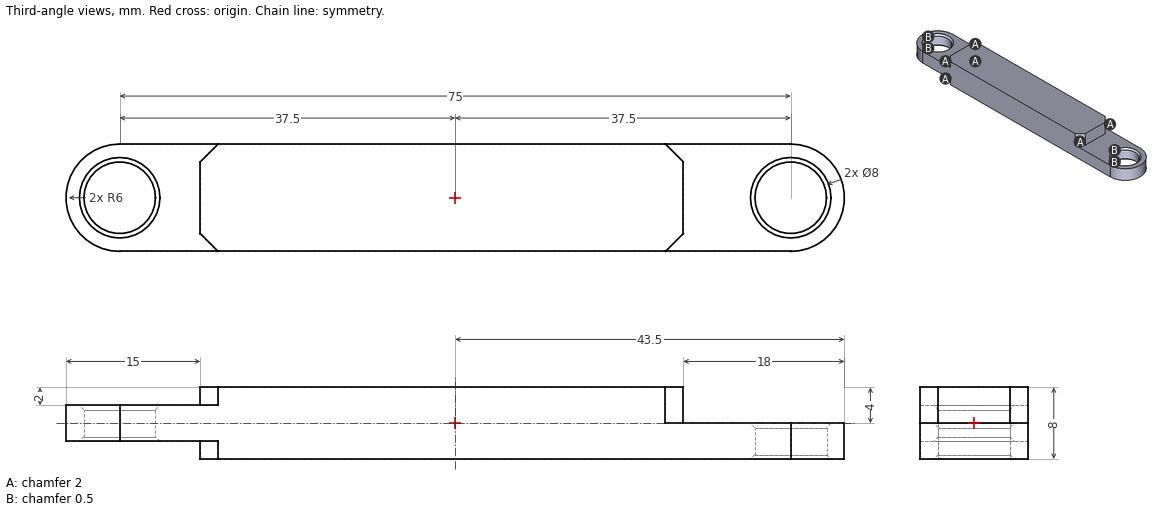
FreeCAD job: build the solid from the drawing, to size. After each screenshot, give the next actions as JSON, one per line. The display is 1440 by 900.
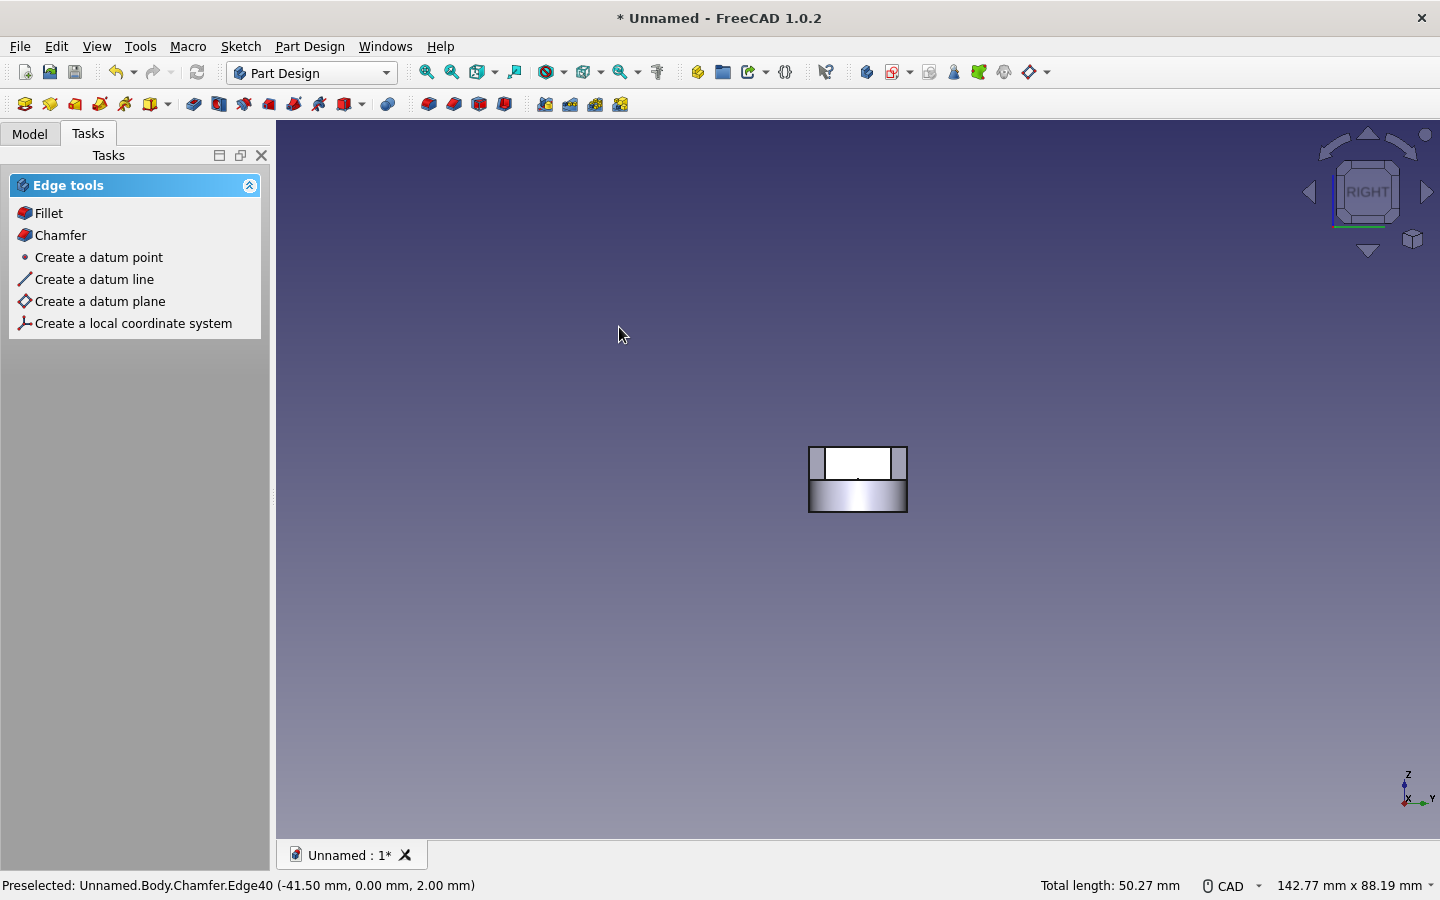
{"action": "left_click", "coordinate": [427, 72]}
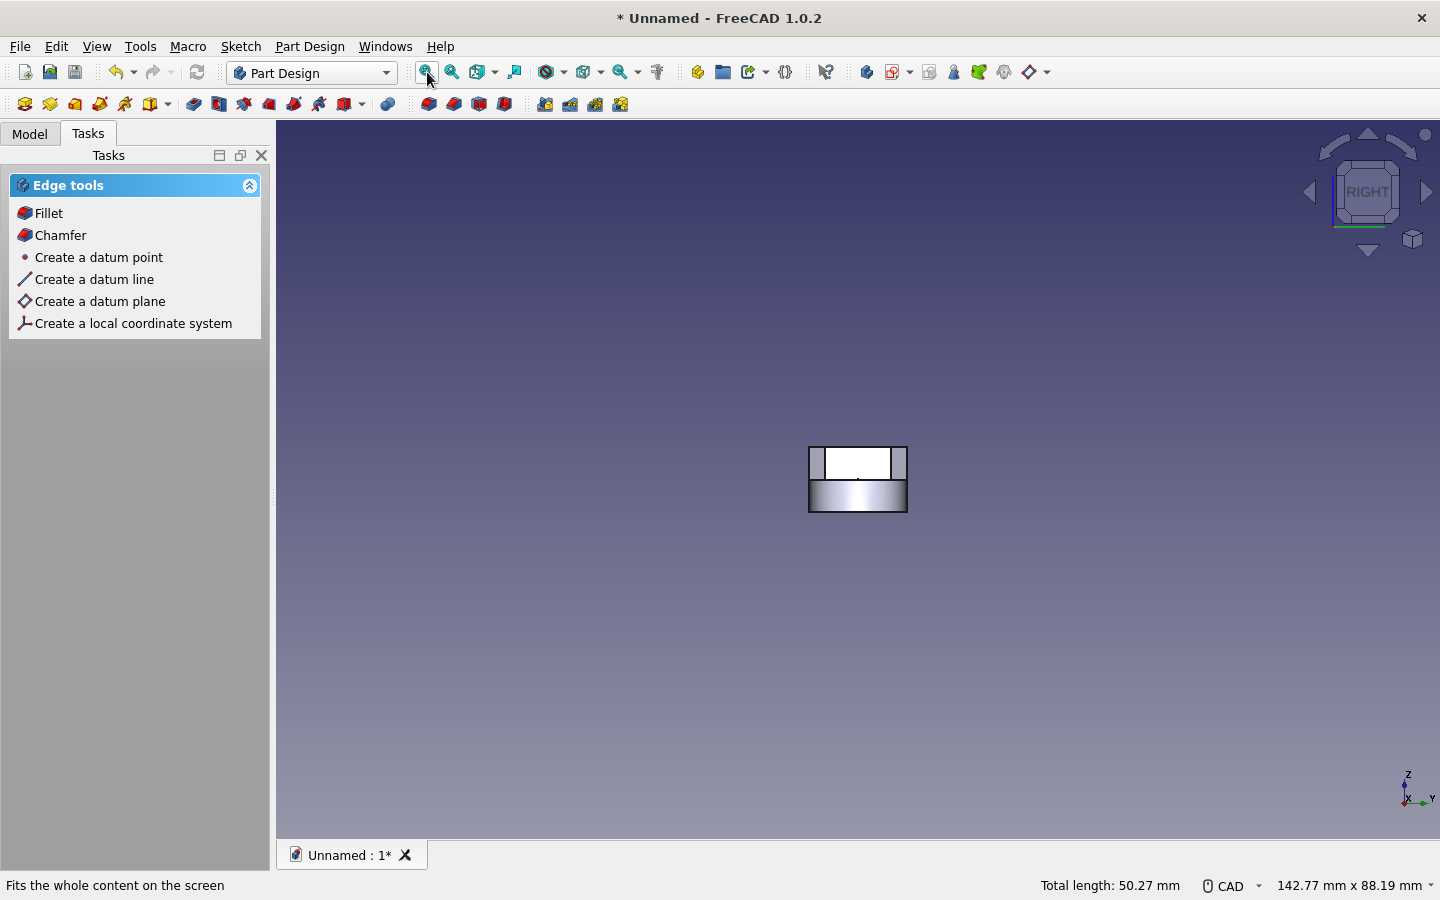
{"action": "key", "text": "5"}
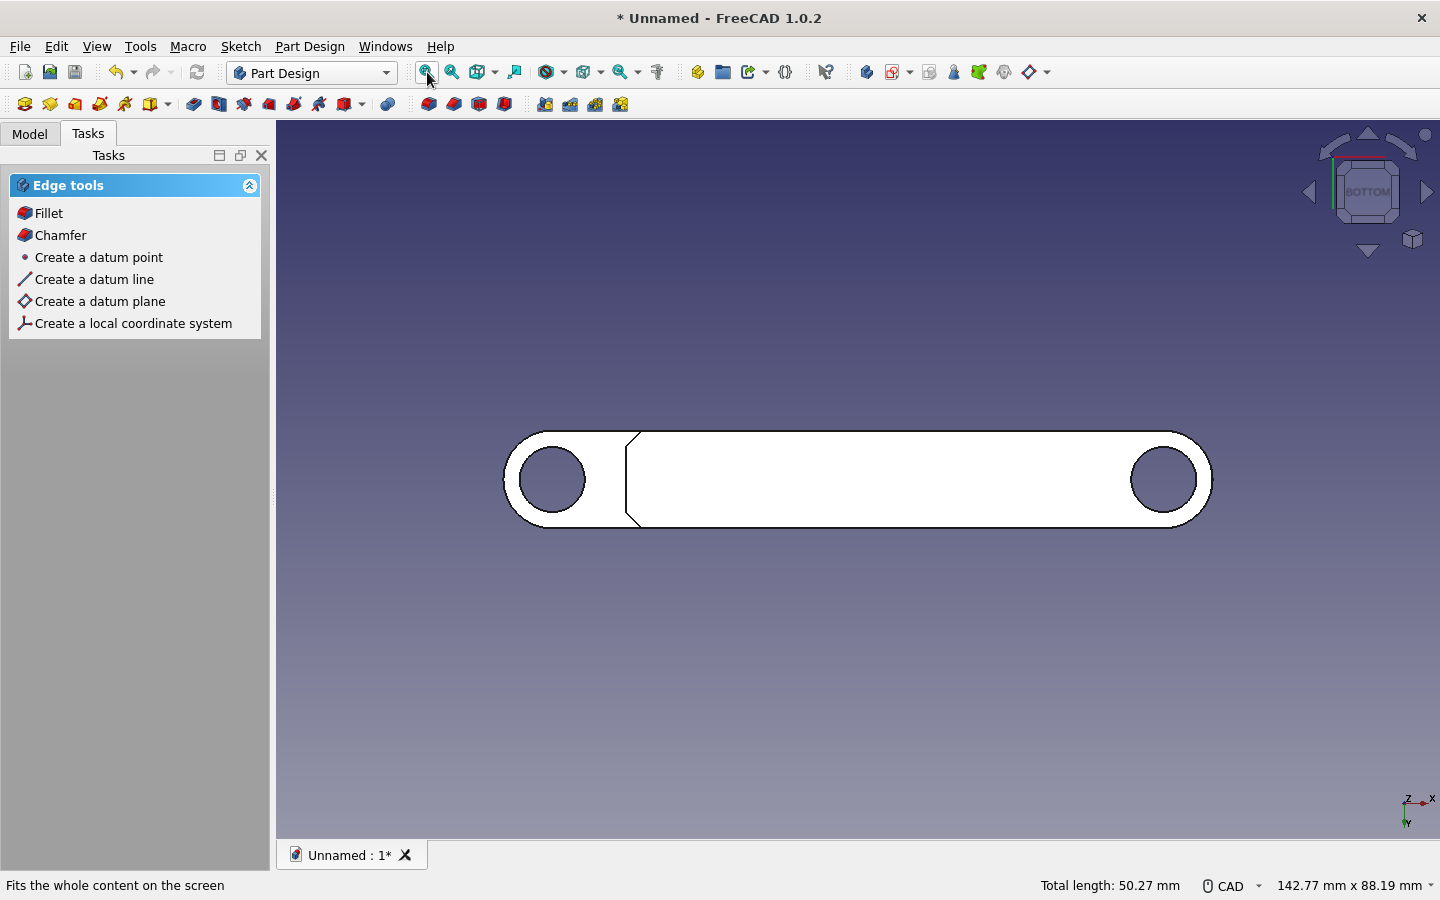
{"action": "left_click", "coordinate": [1131, 478], "text": "ctrl"}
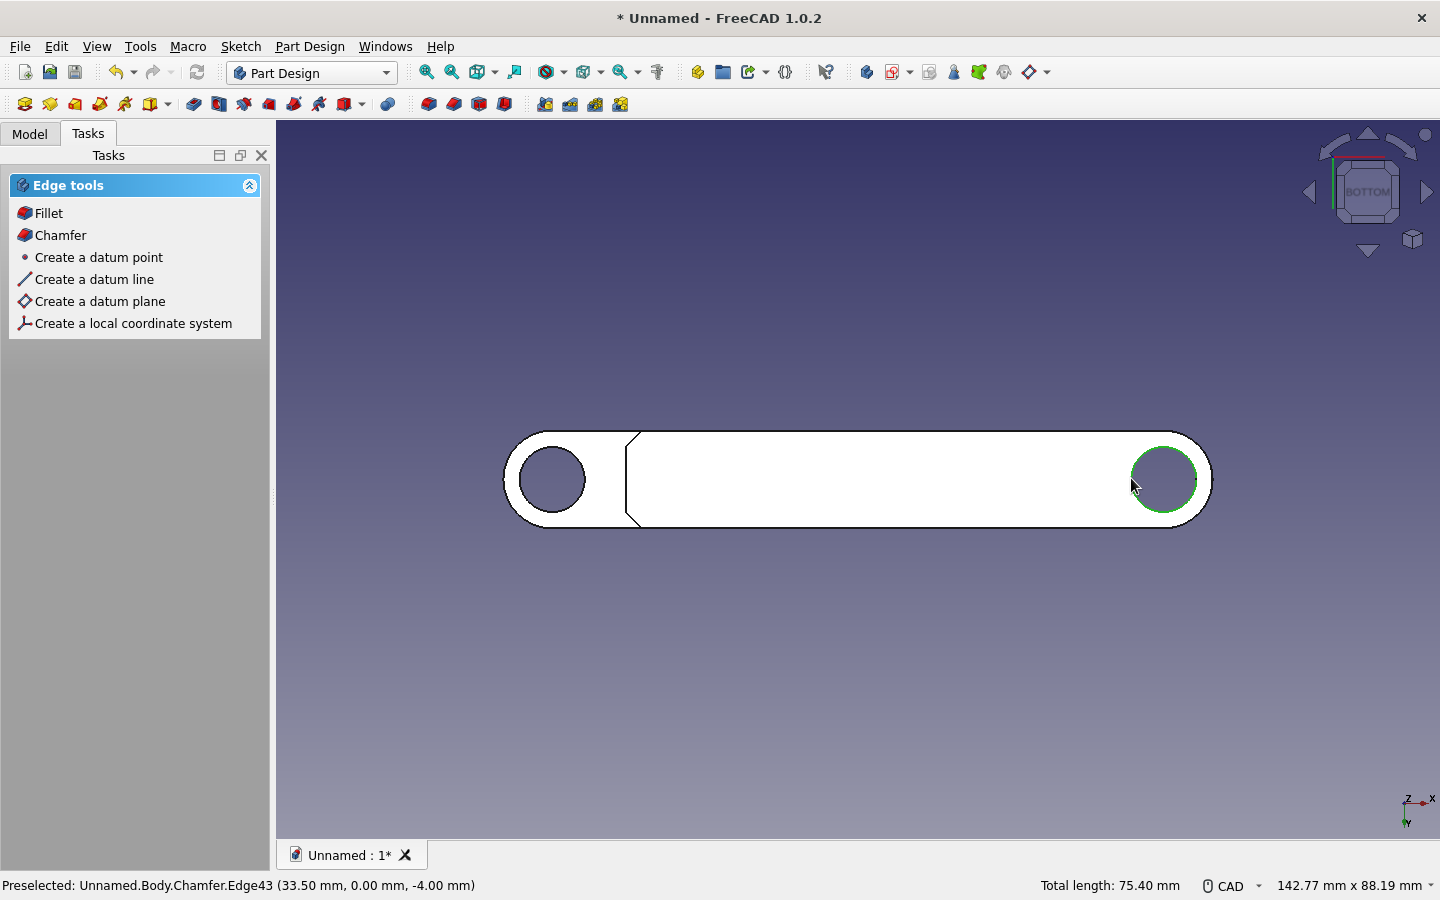
{"action": "left_click", "coordinate": [520, 478], "text": "ctrl"}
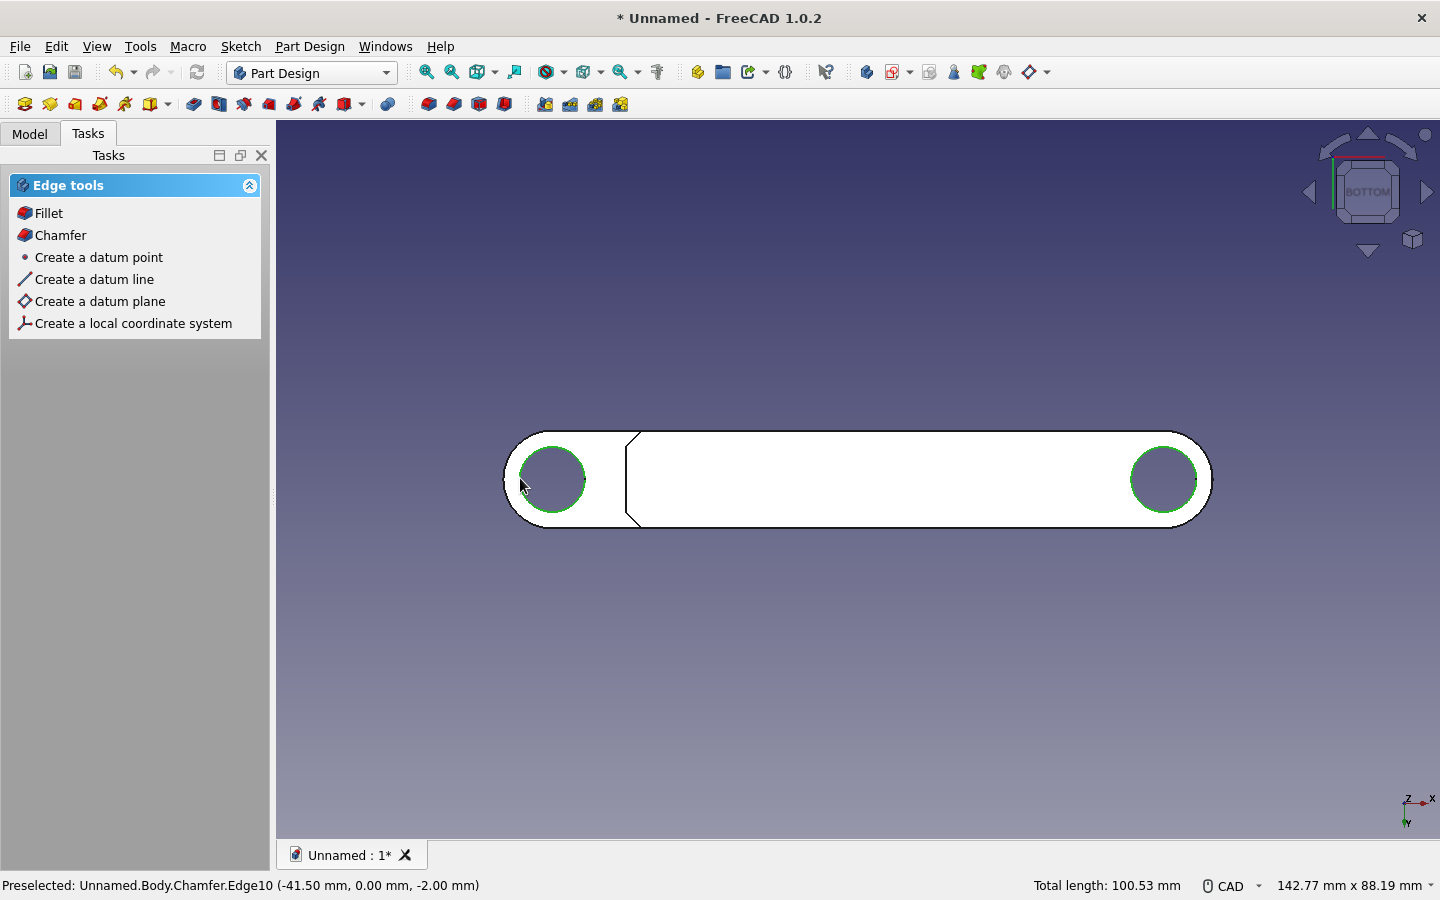
{"action": "left_click", "coordinate": [454, 104]}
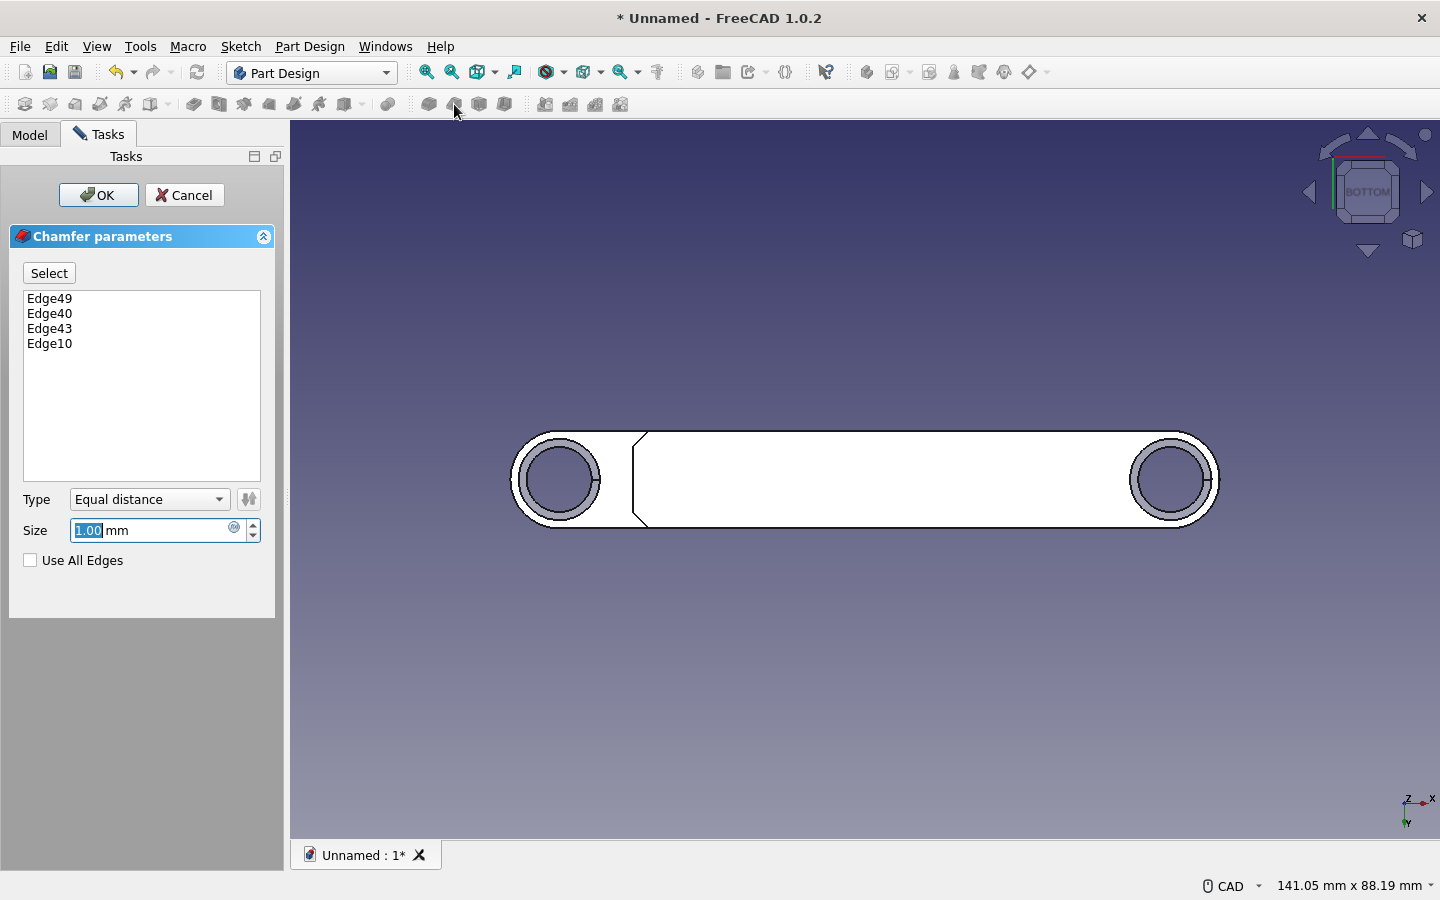
{"action": "type", "text": "0.5"}
{"action": "key", "text": "Tab"}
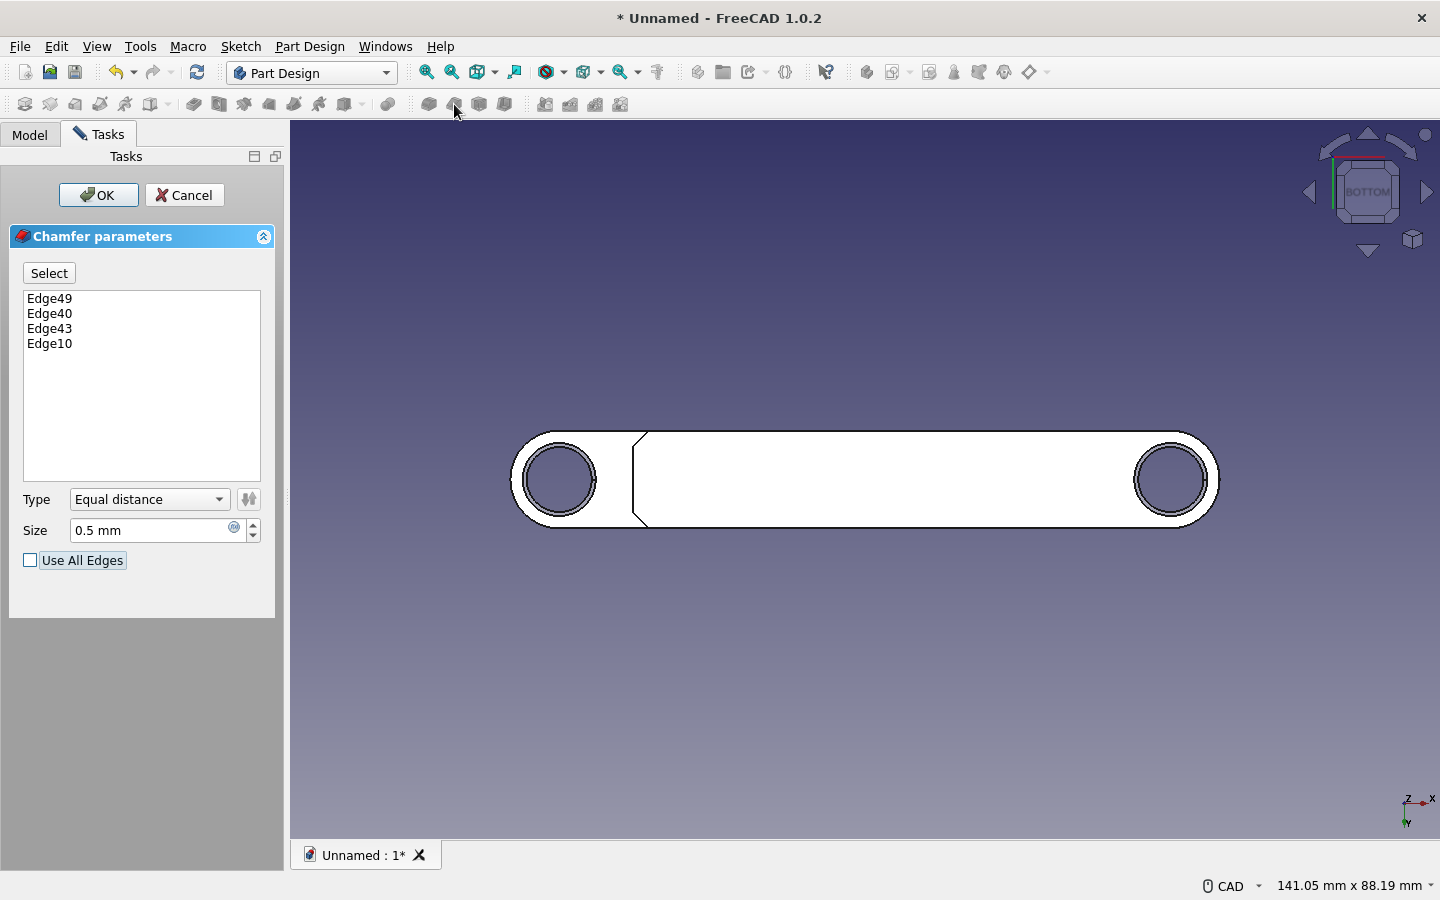
{"action": "left_click", "coordinate": [99, 195]}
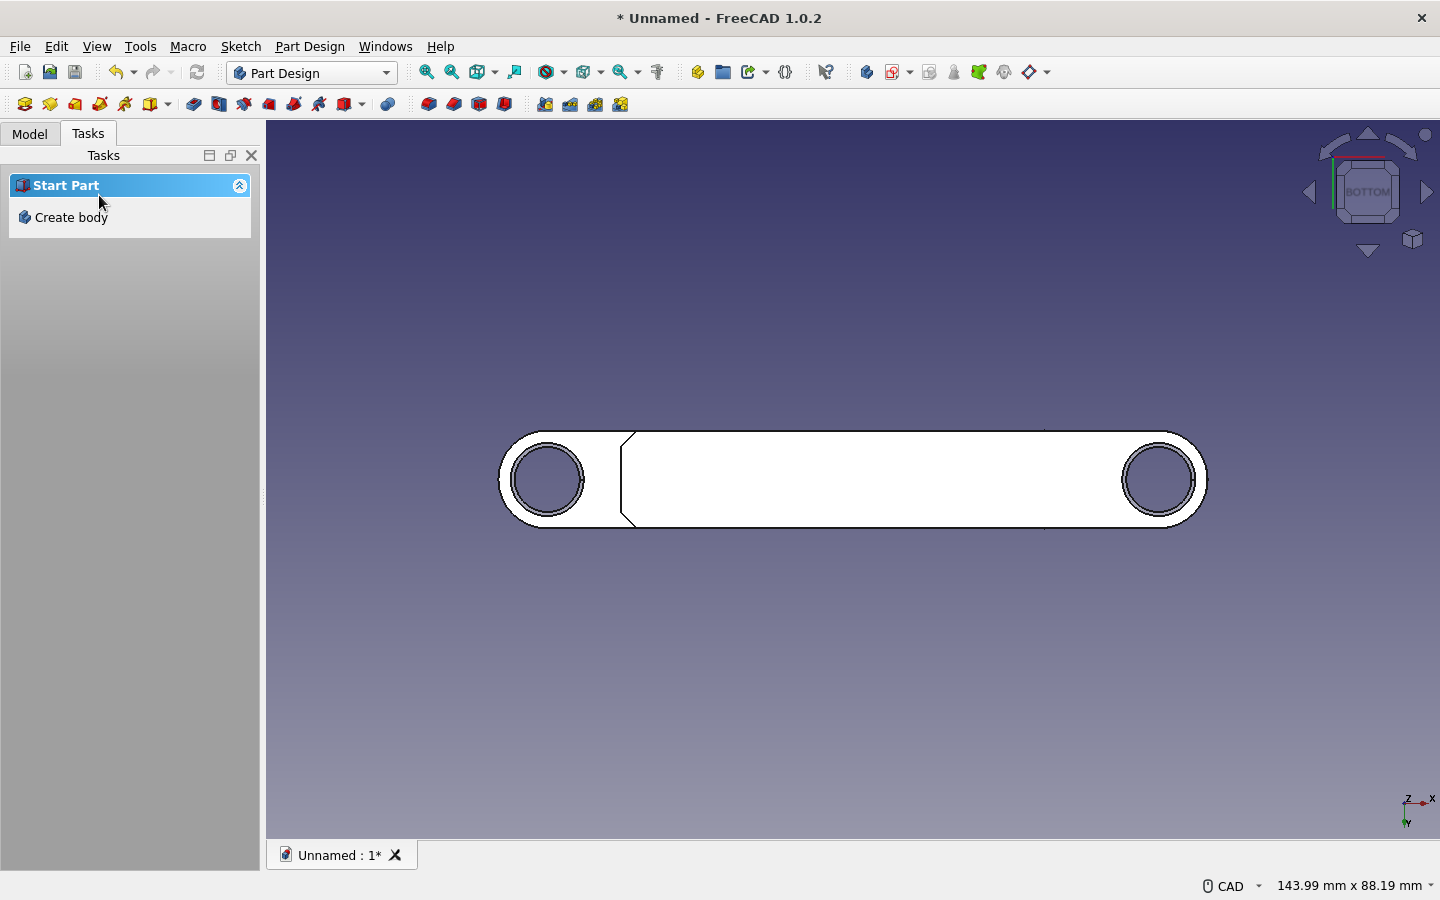
{"action": "key", "text": "0"}